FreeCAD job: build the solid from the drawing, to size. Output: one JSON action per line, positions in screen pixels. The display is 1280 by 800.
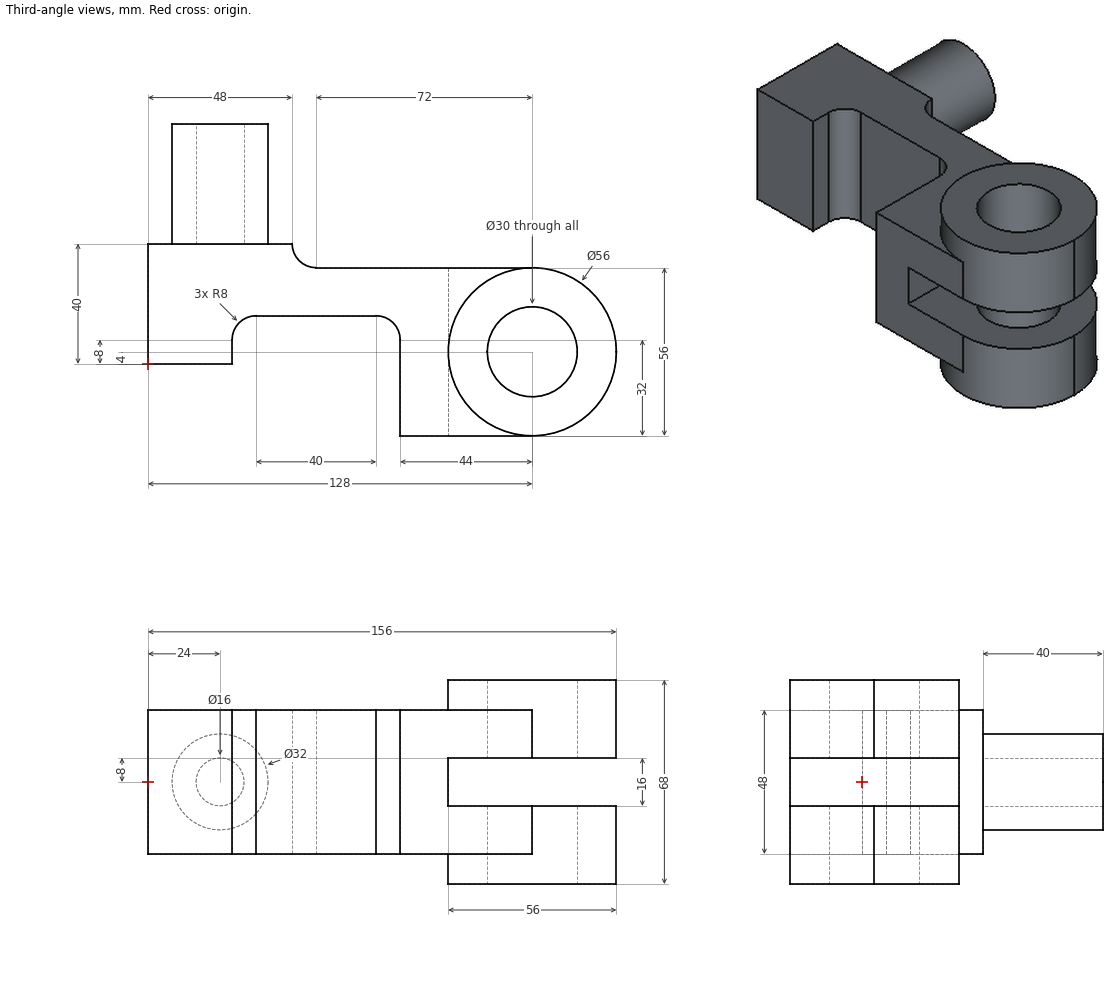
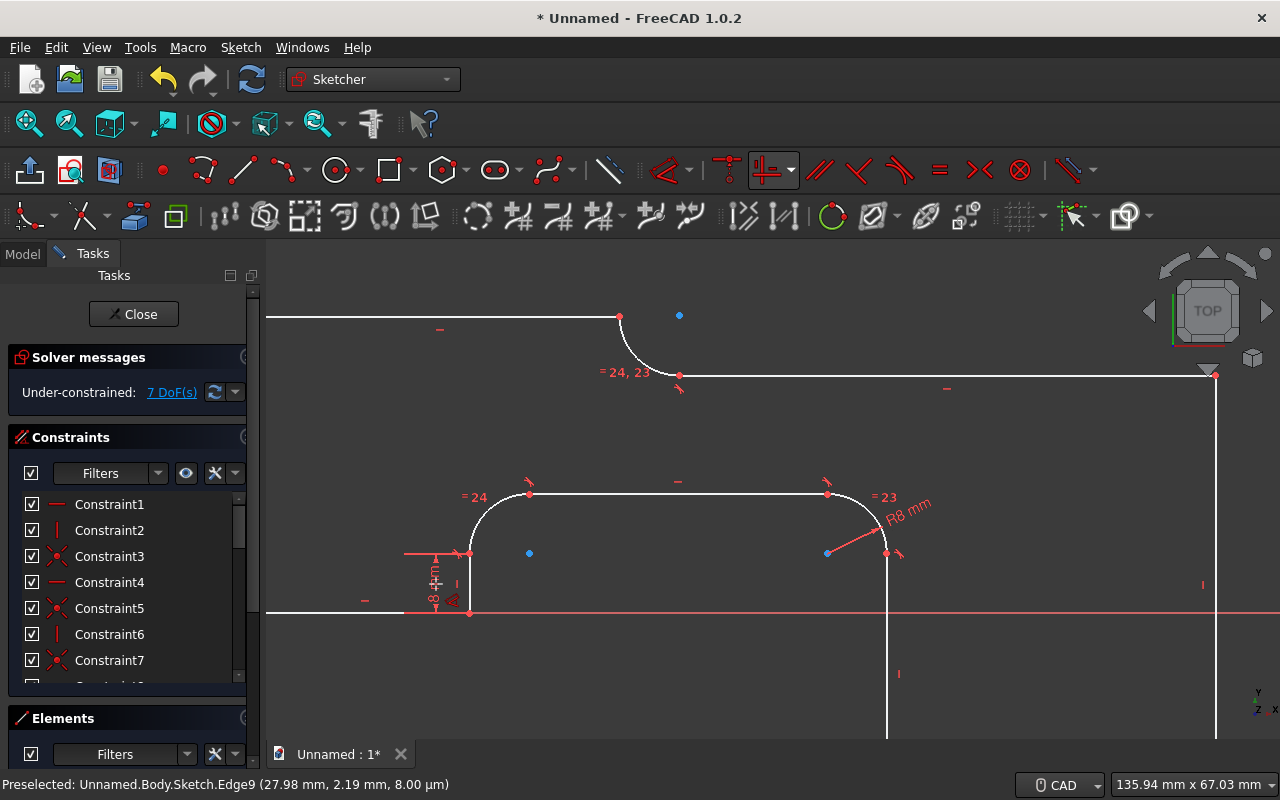
{"action": "left_click", "coordinate": [619, 494]}
{"action": "left_click", "coordinate": [678, 460]}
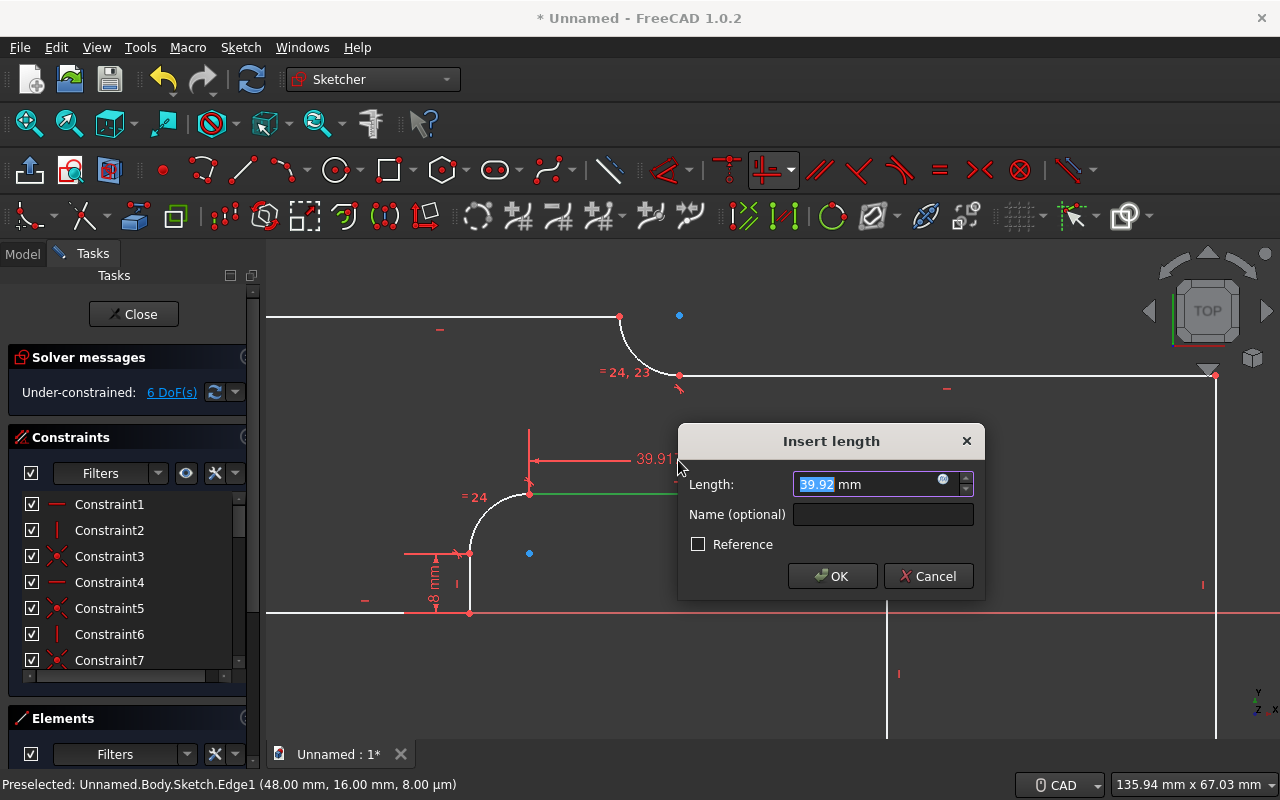
{"action": "type", "text": "40"}
{"action": "key", "text": "Return"}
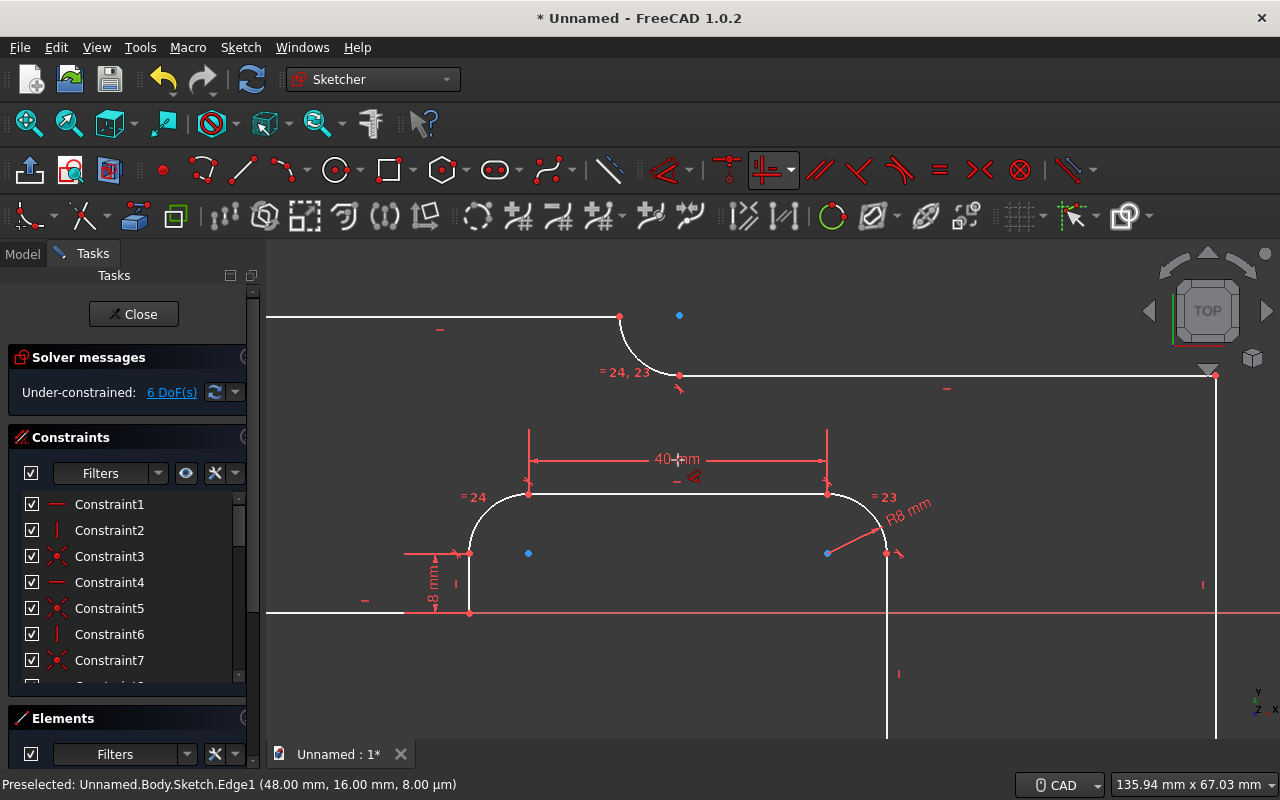
{"action": "left_click", "coordinate": [887, 626]}
{"action": "left_click", "coordinate": [921, 632]}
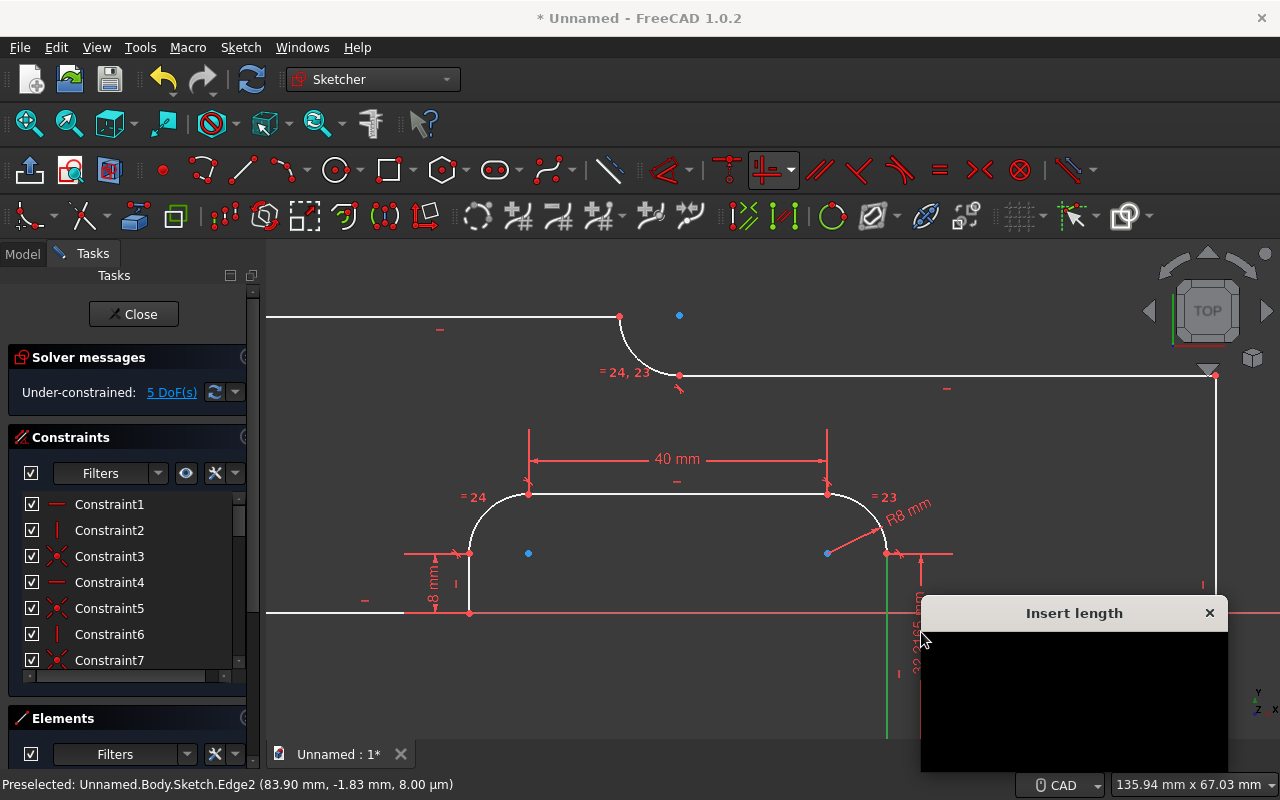
{"action": "type", "text": "32"}
{"action": "key", "text": "Return"}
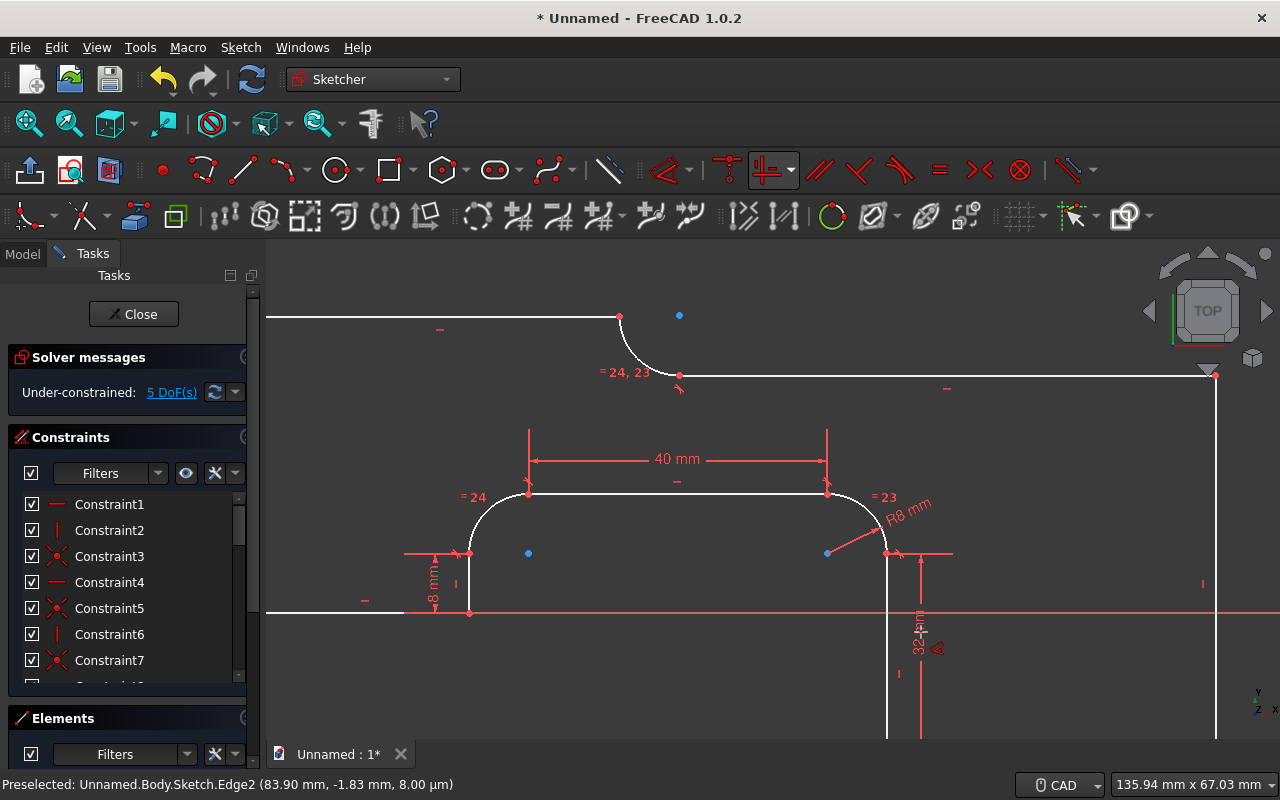
{"action": "scroll", "coordinate": [636, 357], "scroll_direction": "down", "scroll_amount": 2}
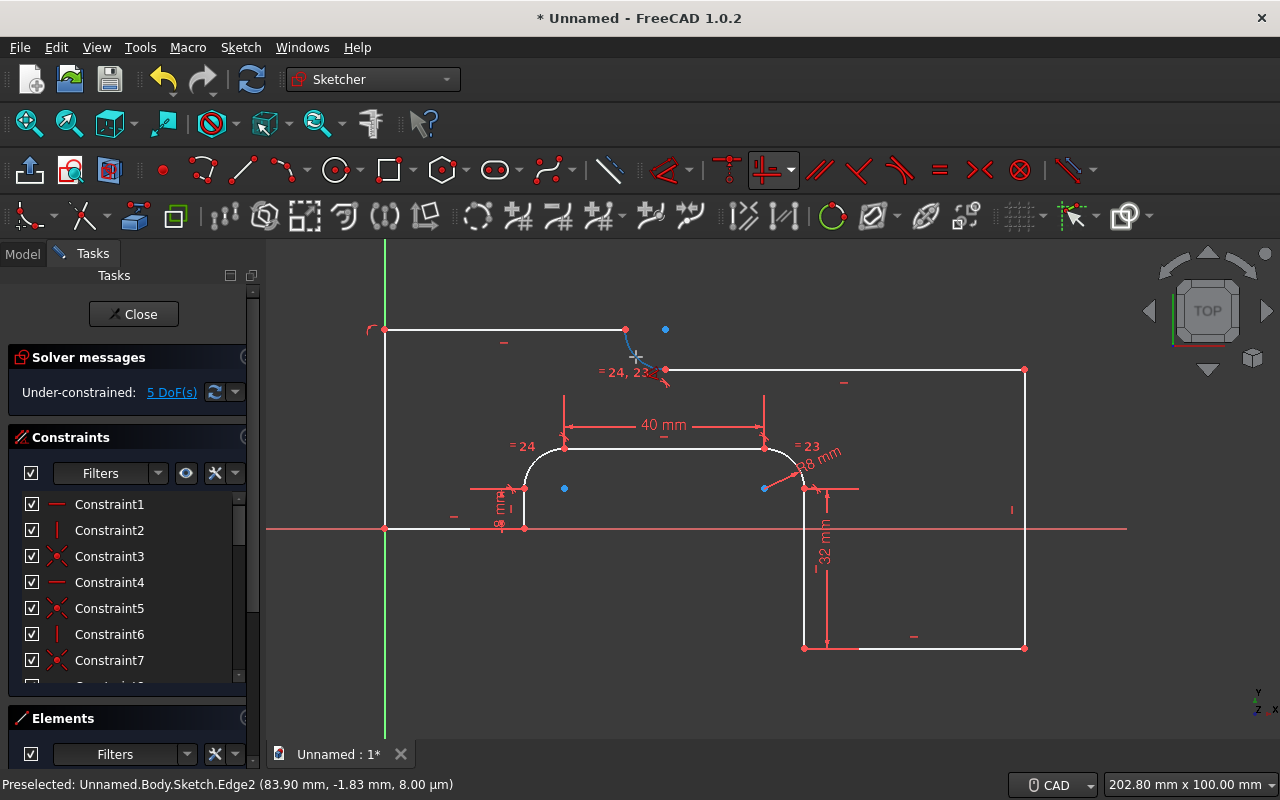
{"action": "left_click", "coordinate": [870, 649]}
{"action": "left_click", "coordinate": [914, 683]}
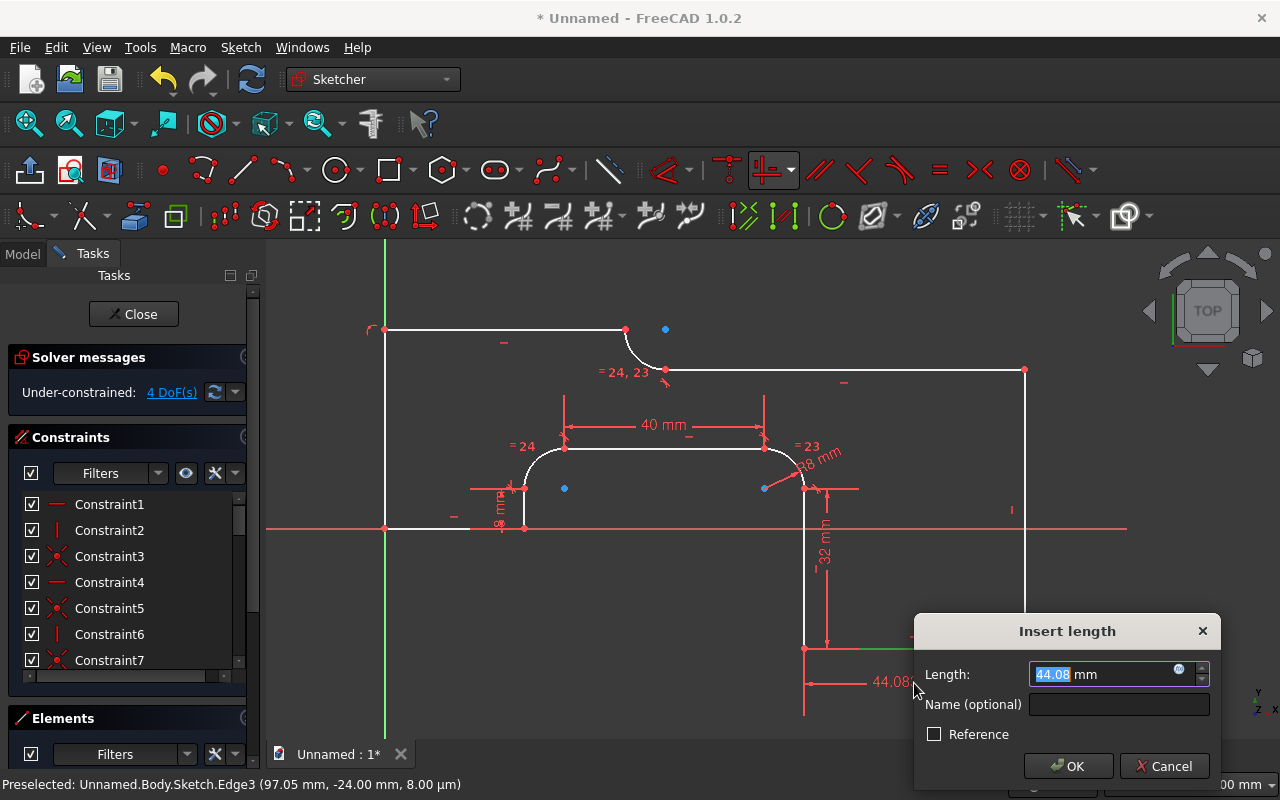
{"action": "type", "text": "44"}
{"action": "key", "text": "Return"}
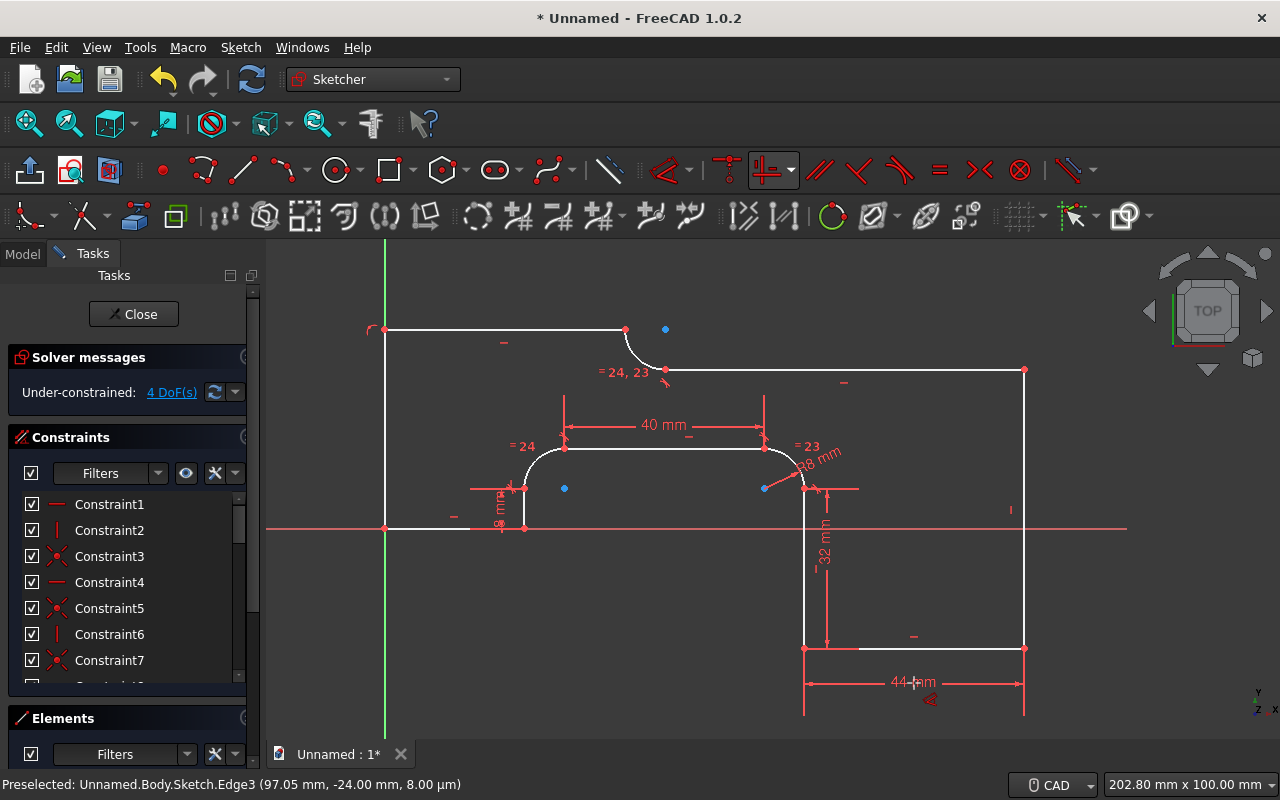
{"action": "left_click", "coordinate": [1024, 565]}
{"action": "left_click", "coordinate": [1058, 509]}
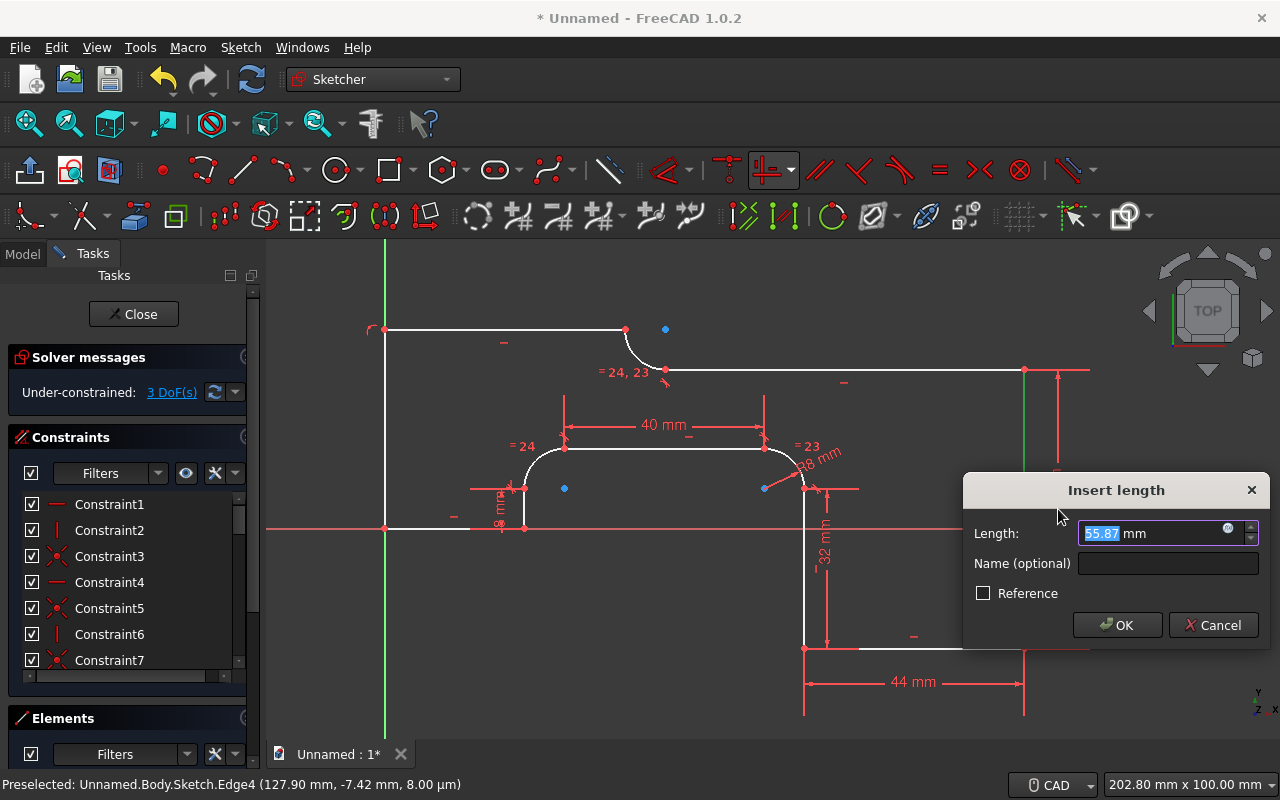
{"action": "type", "text": "56"}
{"action": "key", "text": "Return"}